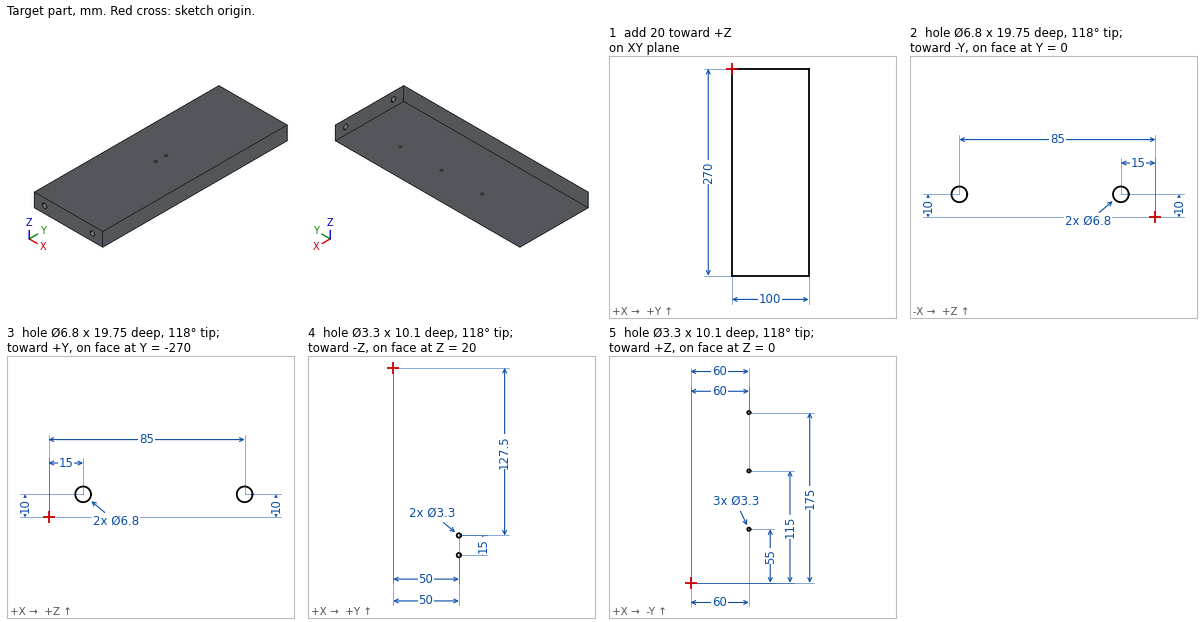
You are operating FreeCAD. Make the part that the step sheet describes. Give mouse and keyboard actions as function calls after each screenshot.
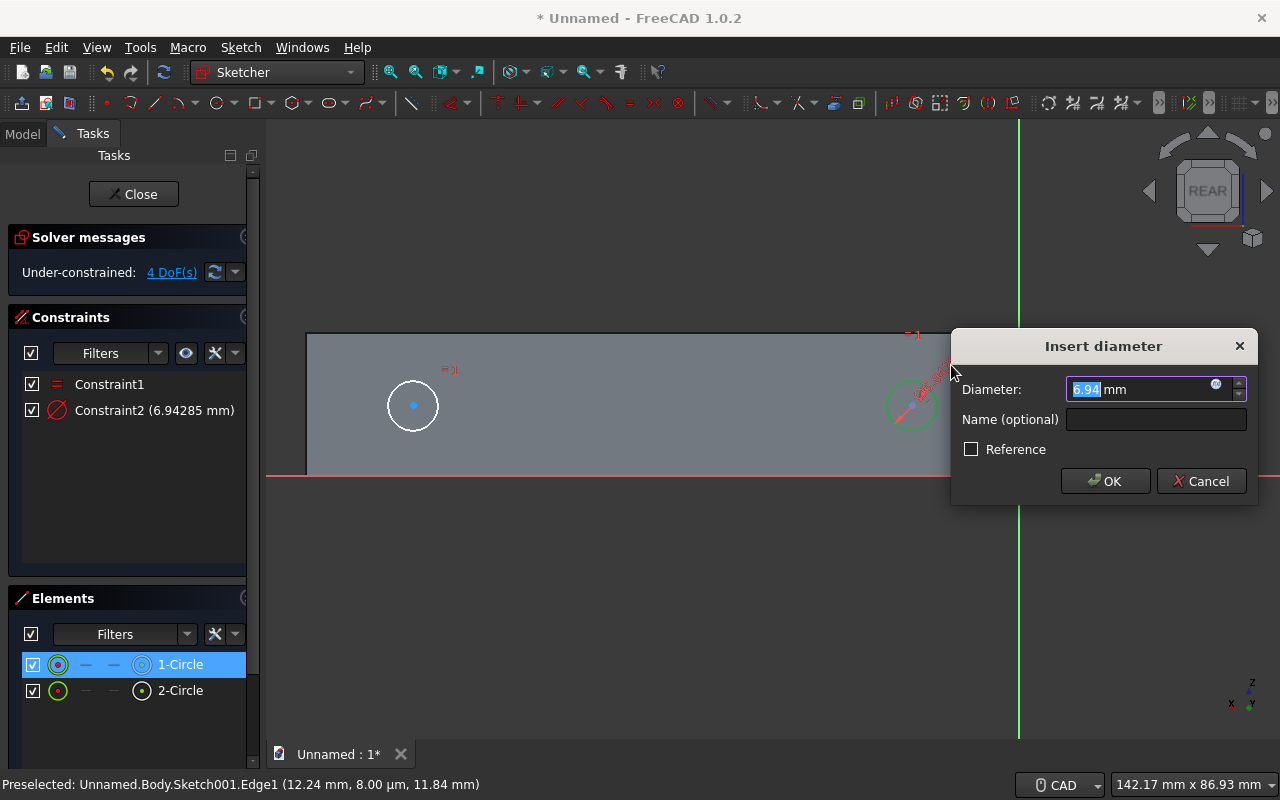
text(6.8)
key(Return)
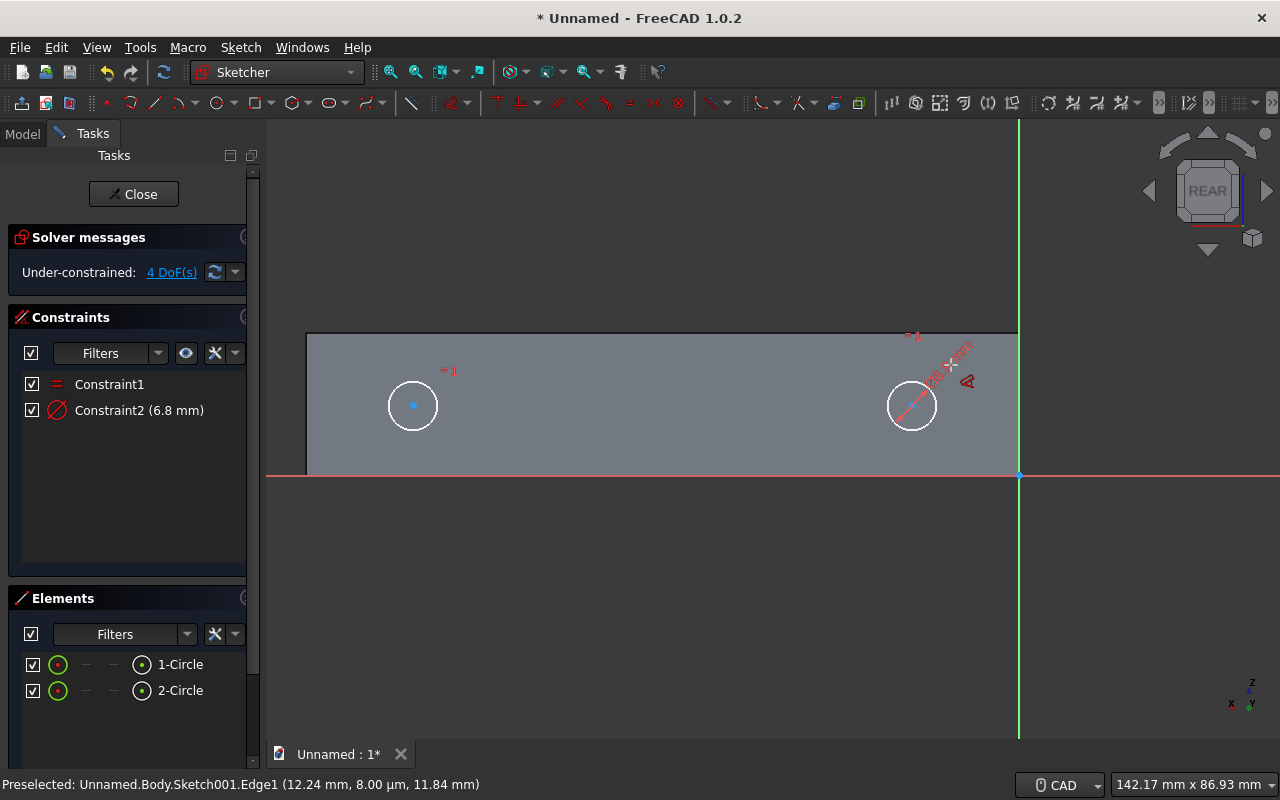
click(912, 406)
click(966, 510)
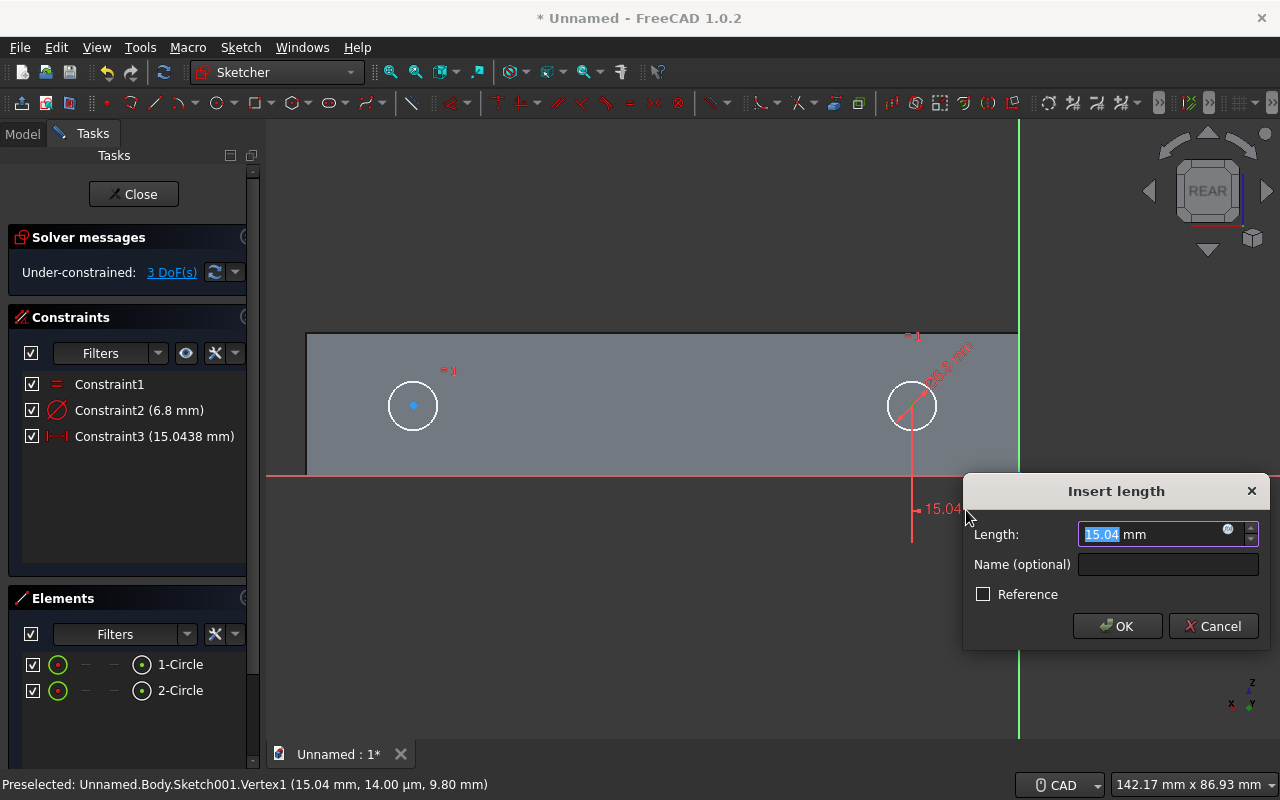
text(15)
key(Return)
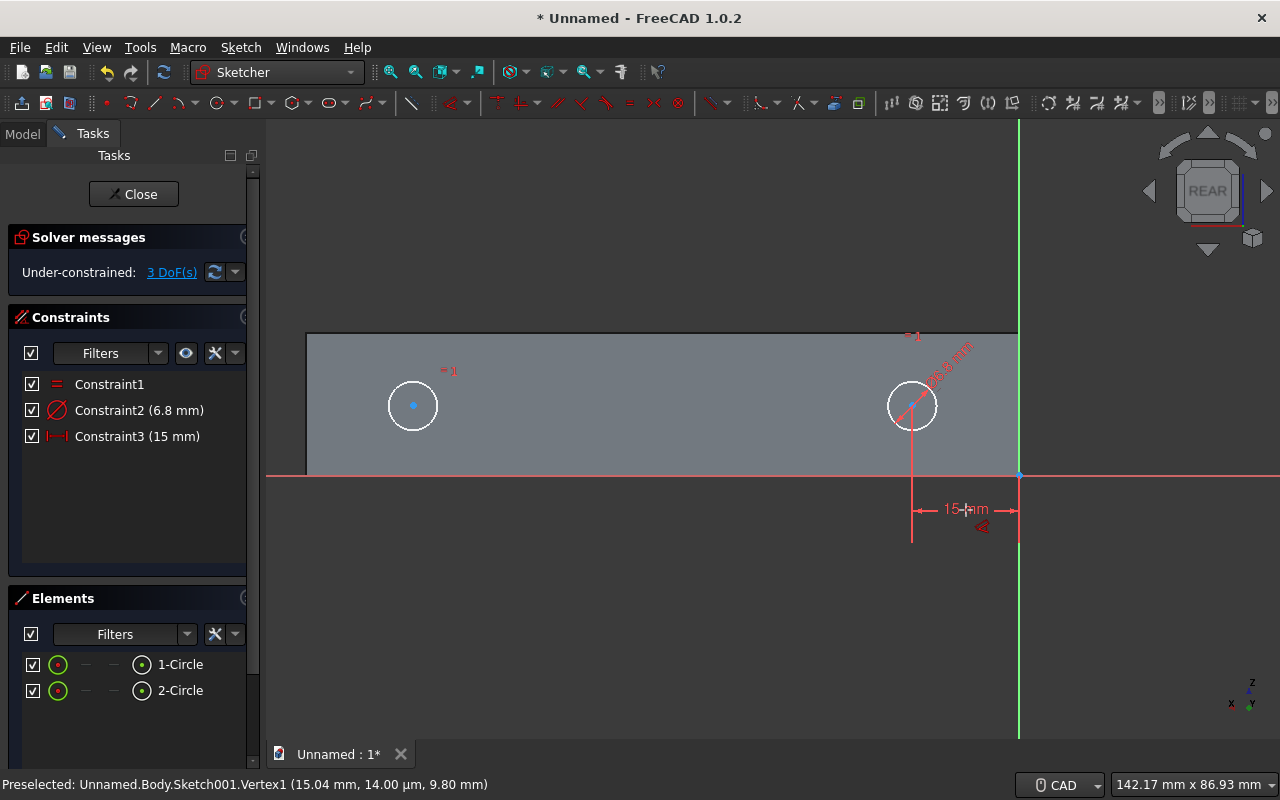
click(912, 406)
click(1053, 441)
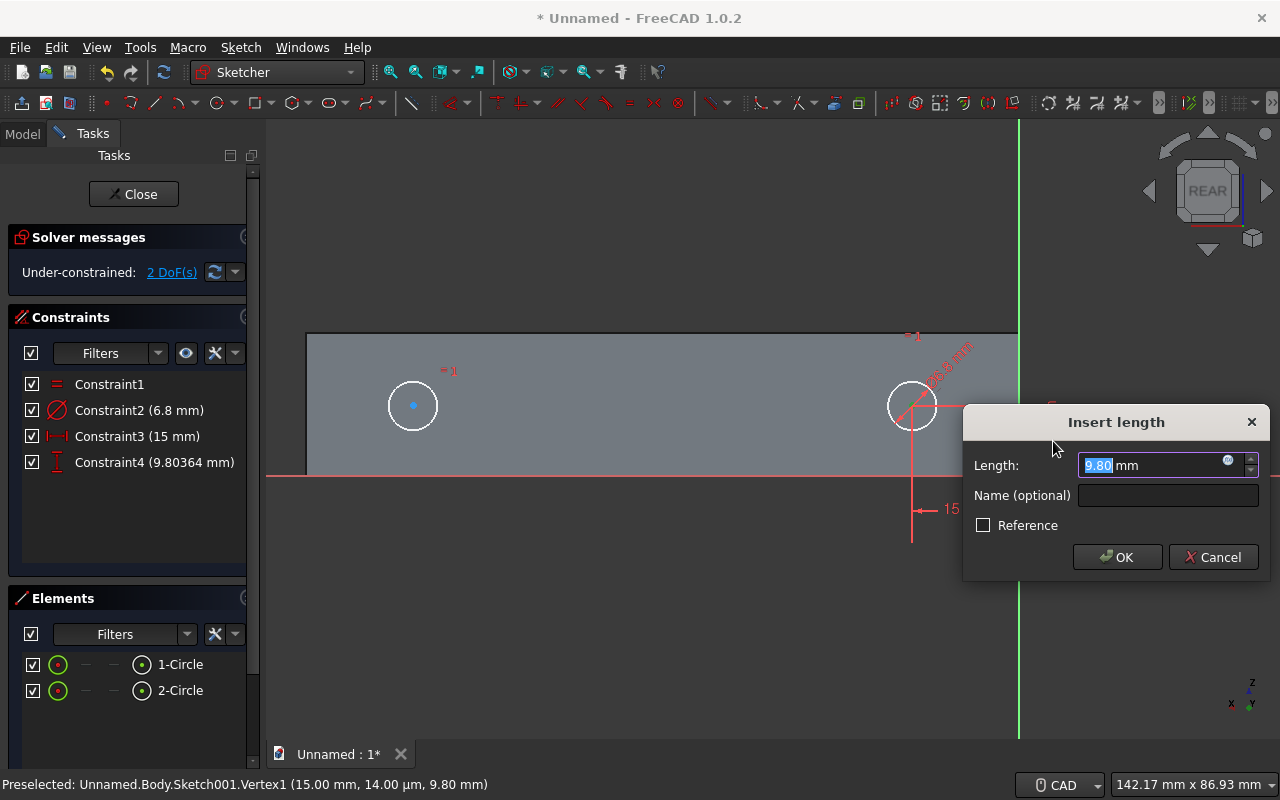
text(10)
key(Return)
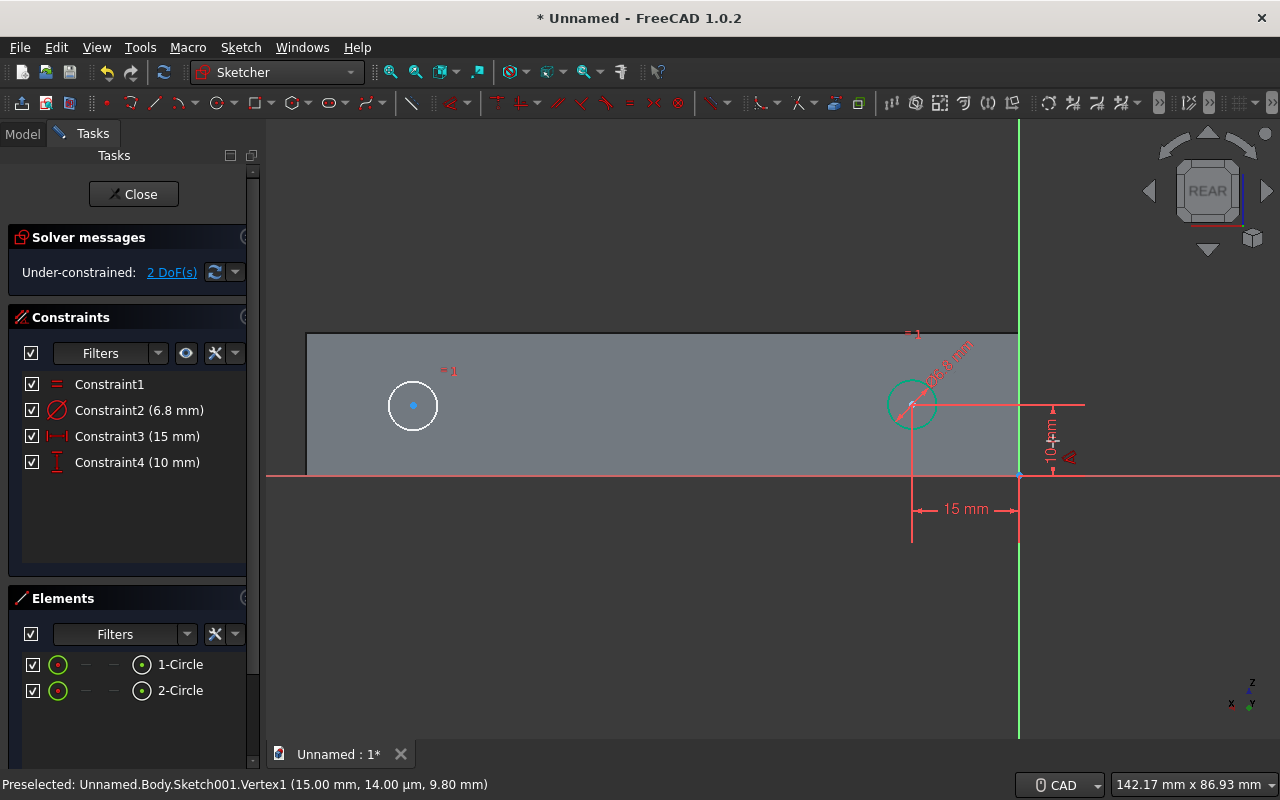
click(413, 406)
click(716, 510)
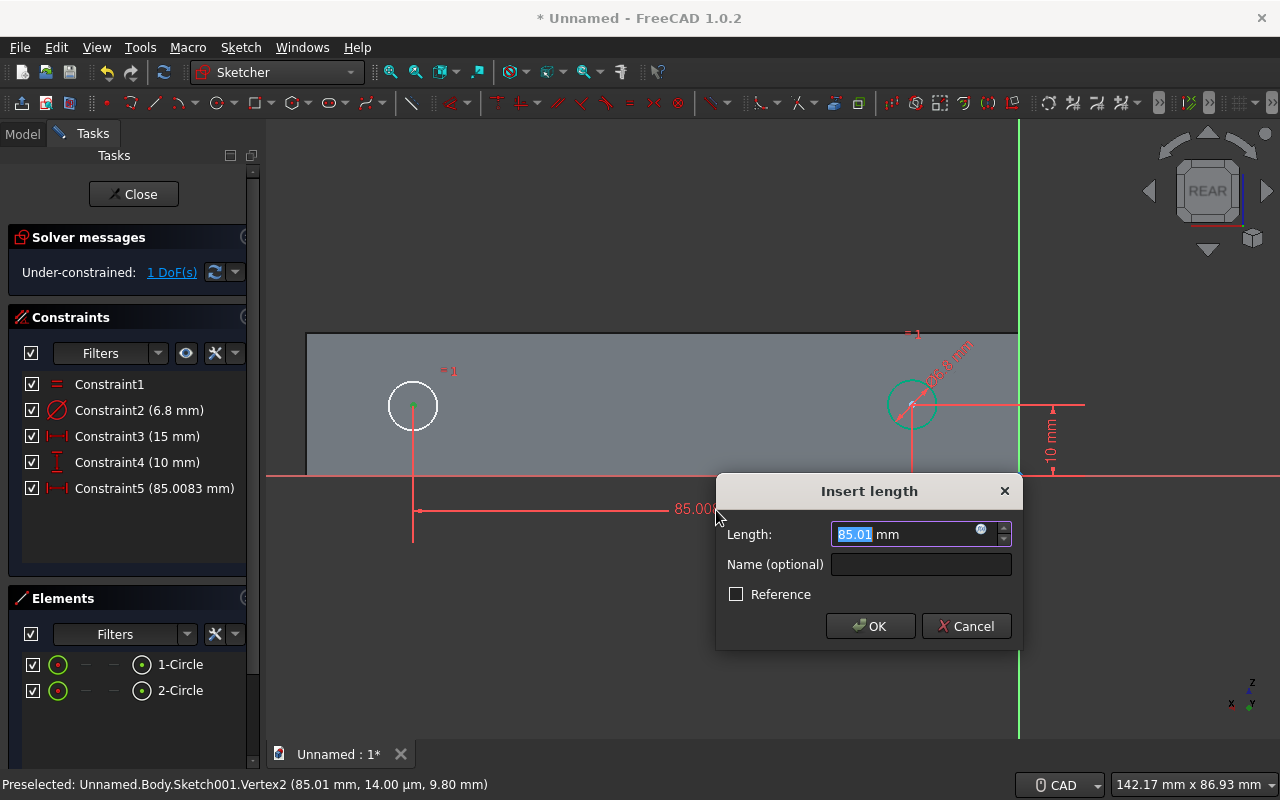
text(85)
key(Return)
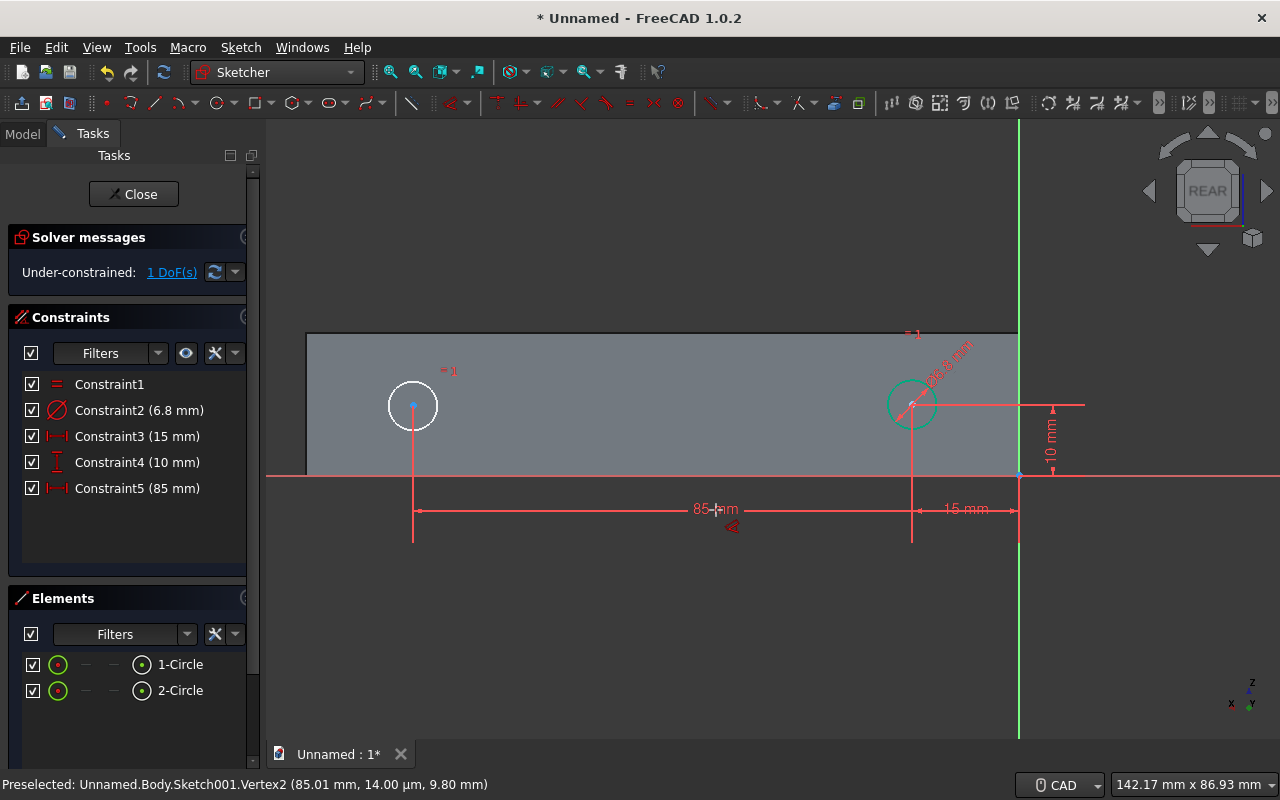
click(413, 406)
click(1053, 416)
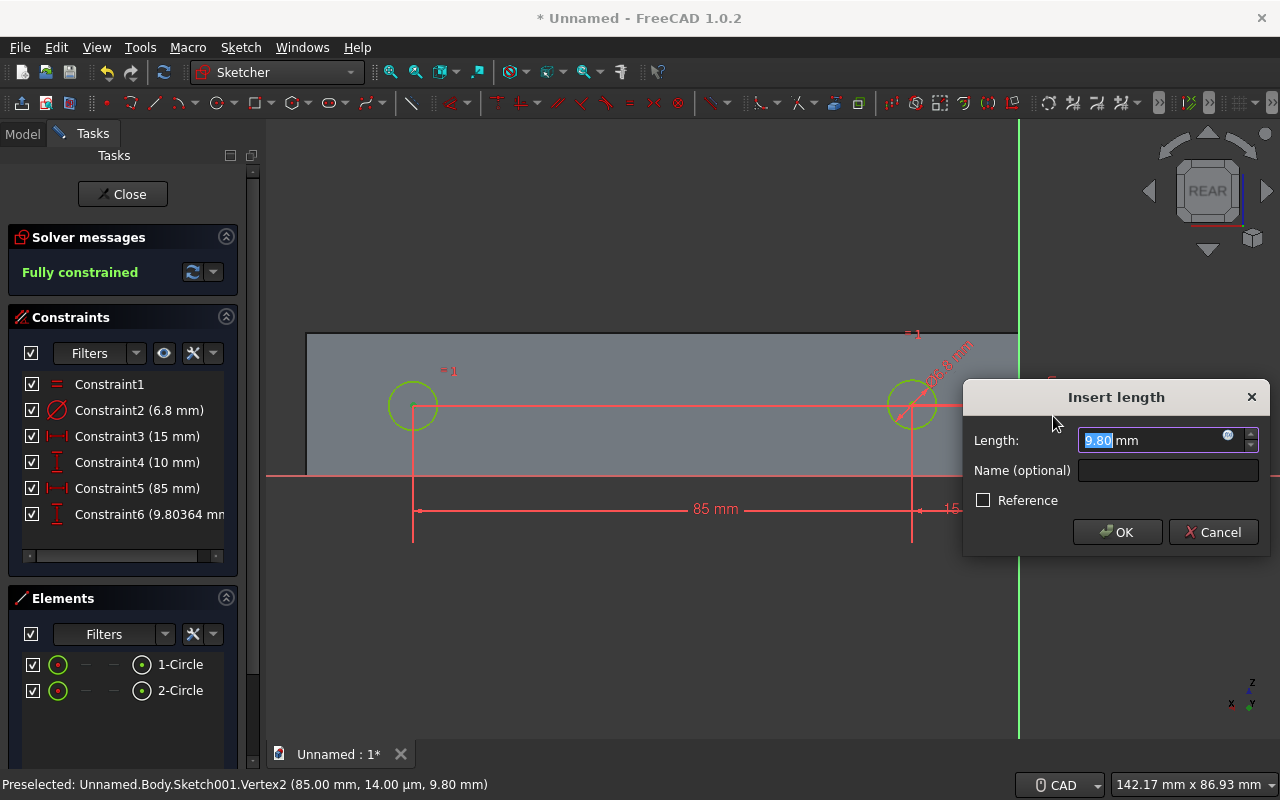
text(10)
key(Return)
key(Escape)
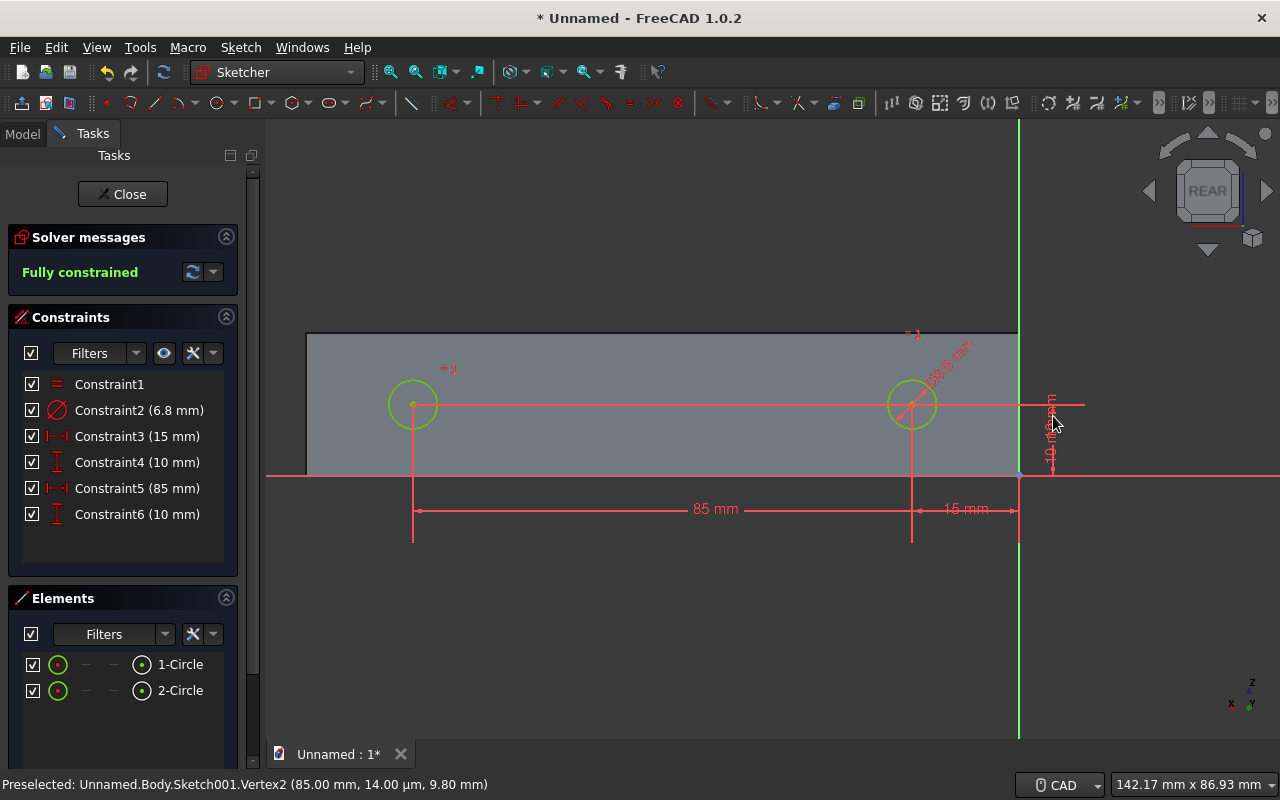
click(123, 194)